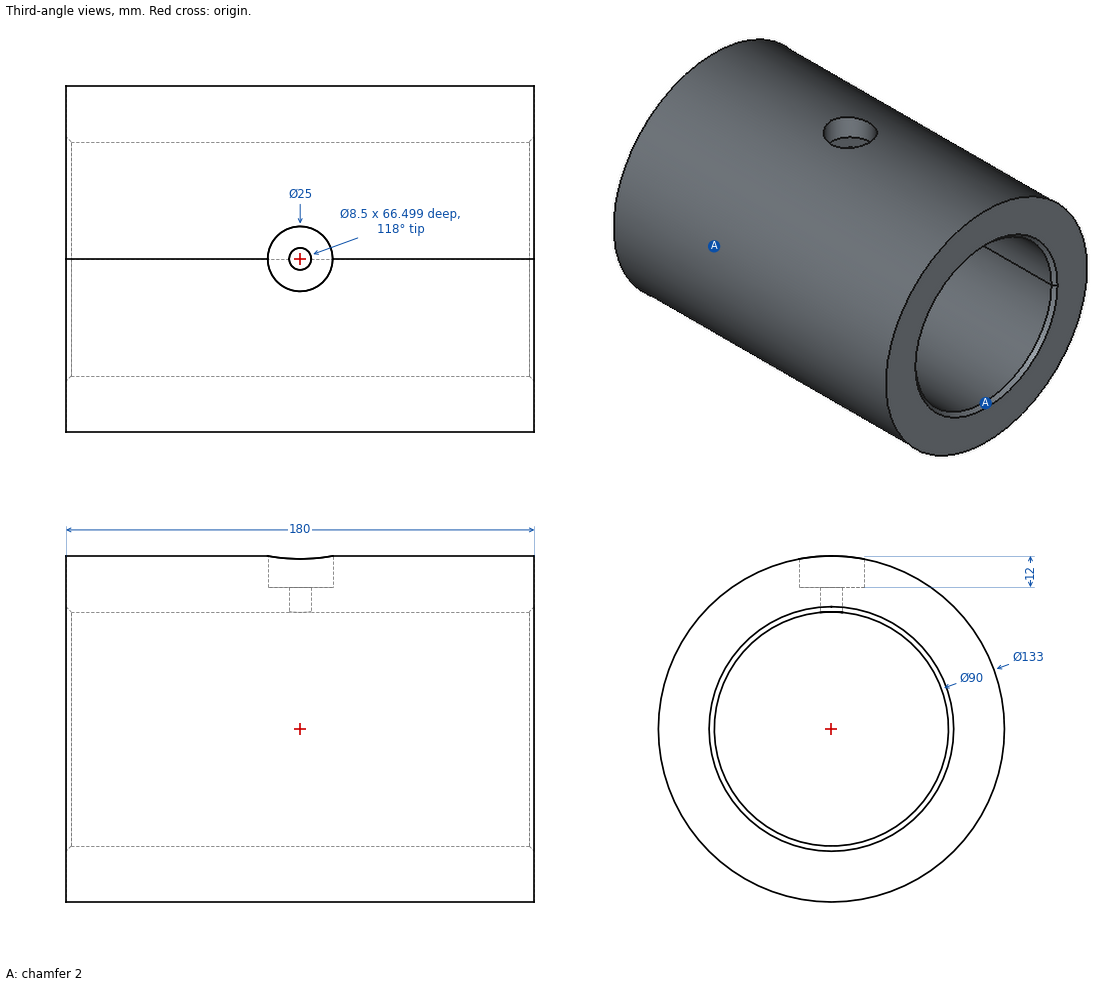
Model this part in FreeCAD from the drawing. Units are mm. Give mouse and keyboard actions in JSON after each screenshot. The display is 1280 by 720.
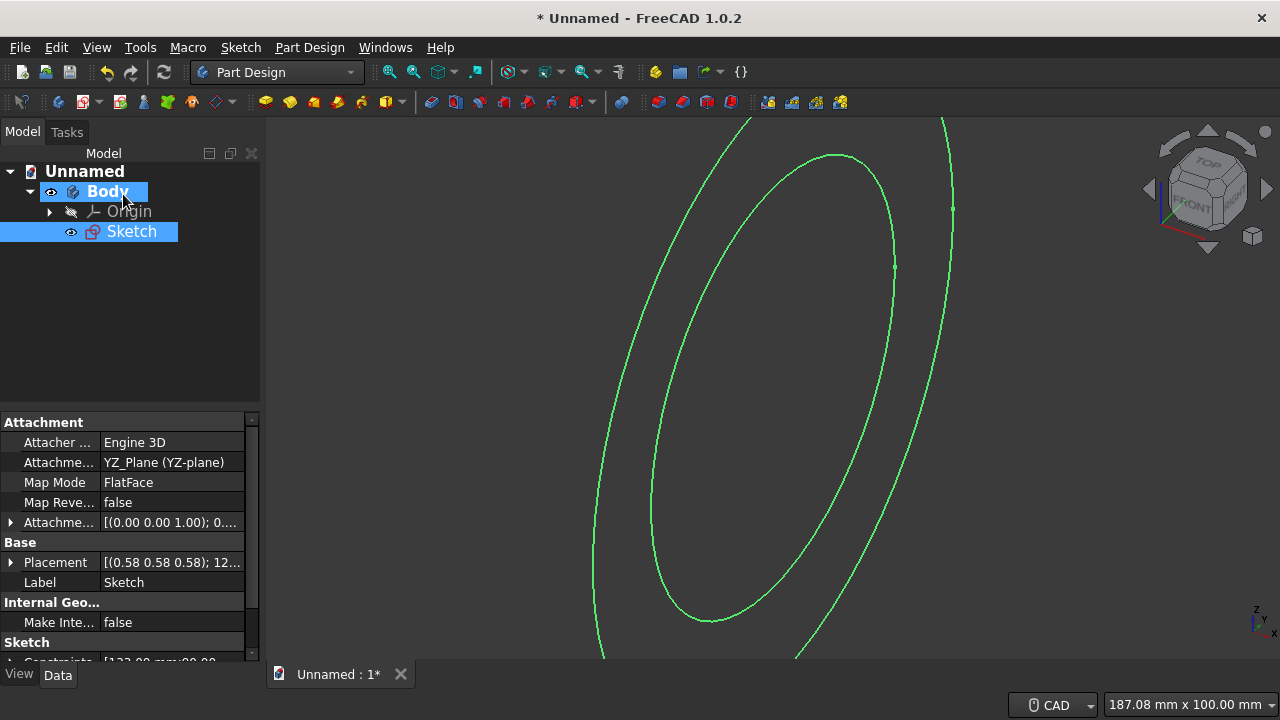
{"action": "left_click", "coordinate": [266, 102]}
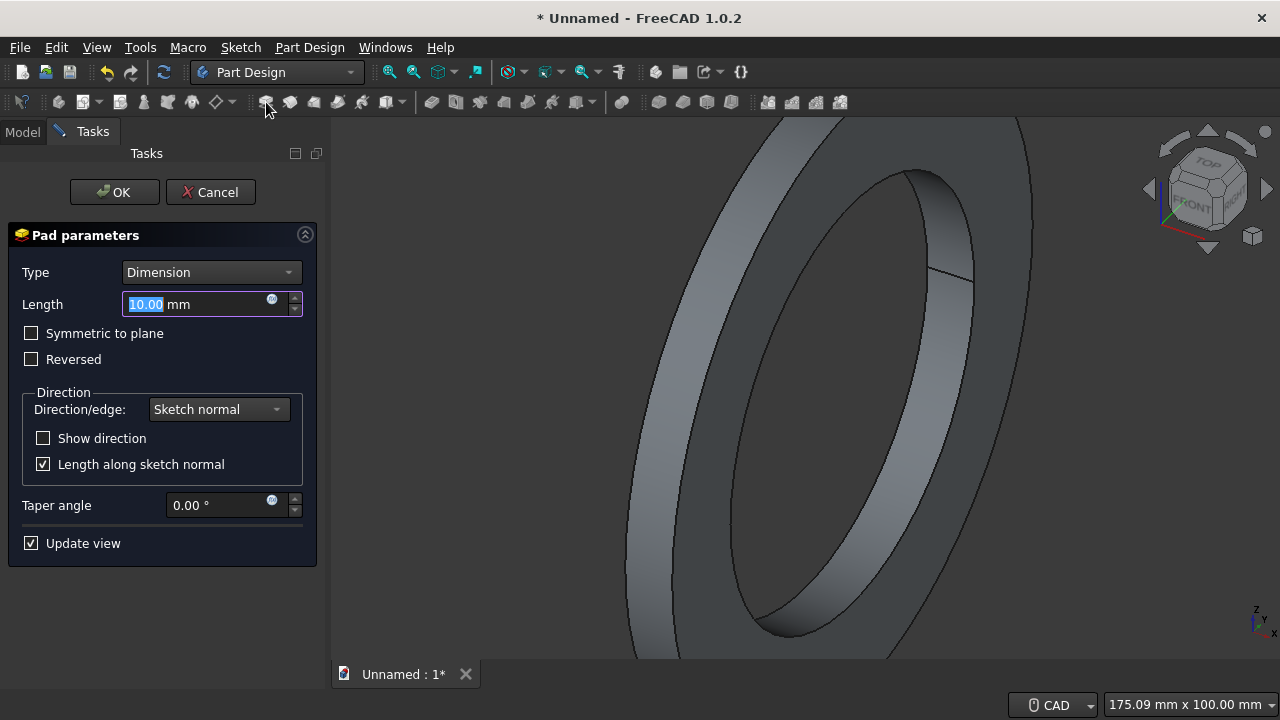
{"action": "type", "text": "180"}
{"action": "key", "text": "Tab"}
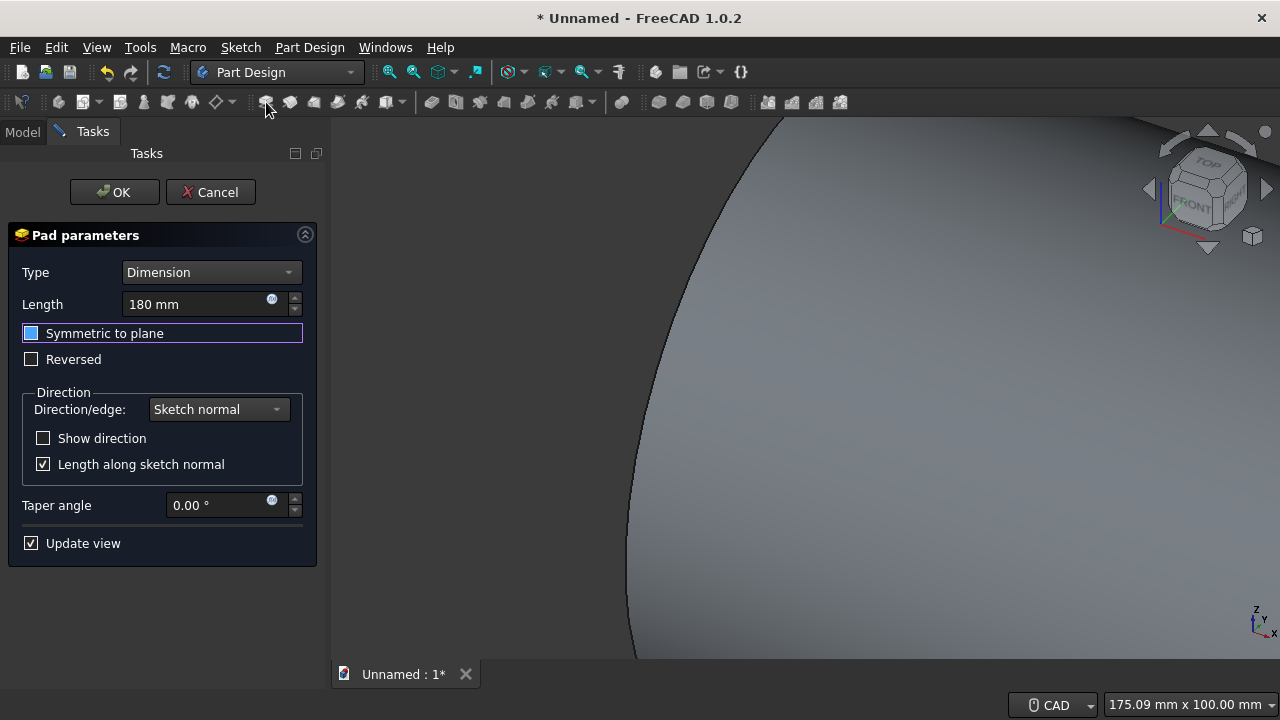
{"action": "left_click", "coordinate": [30, 333]}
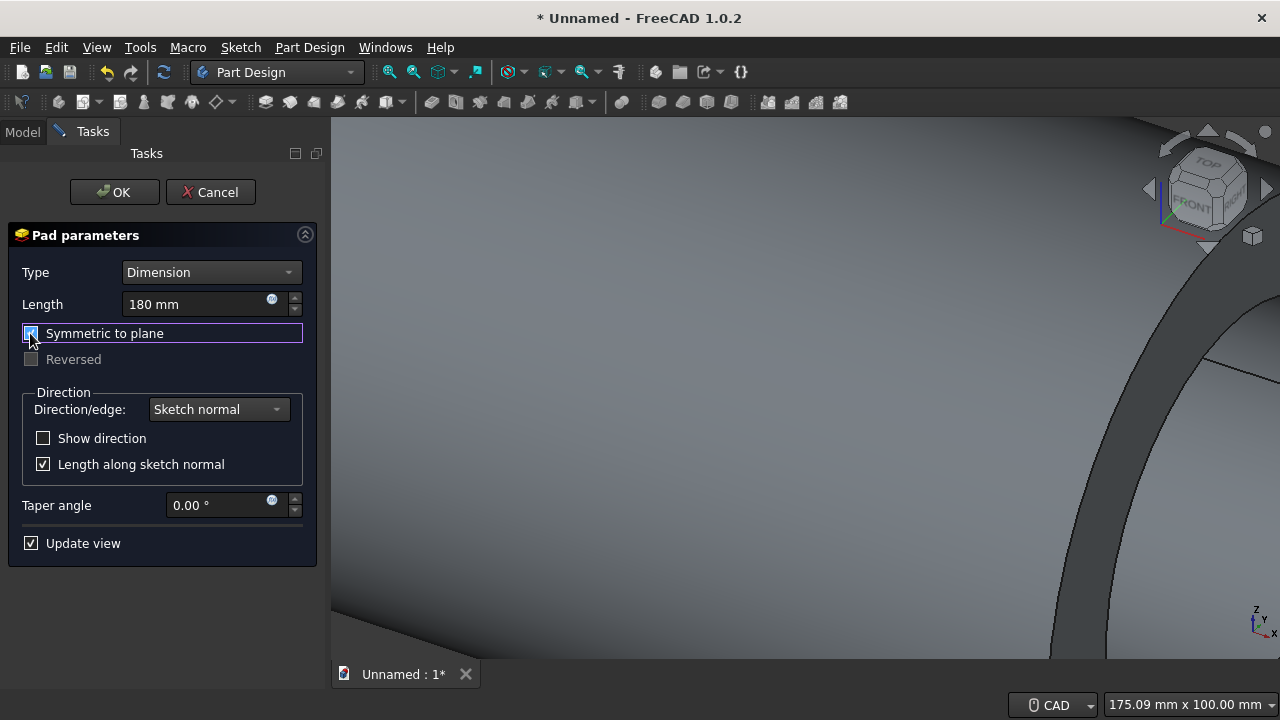
{"action": "left_click", "coordinate": [115, 192]}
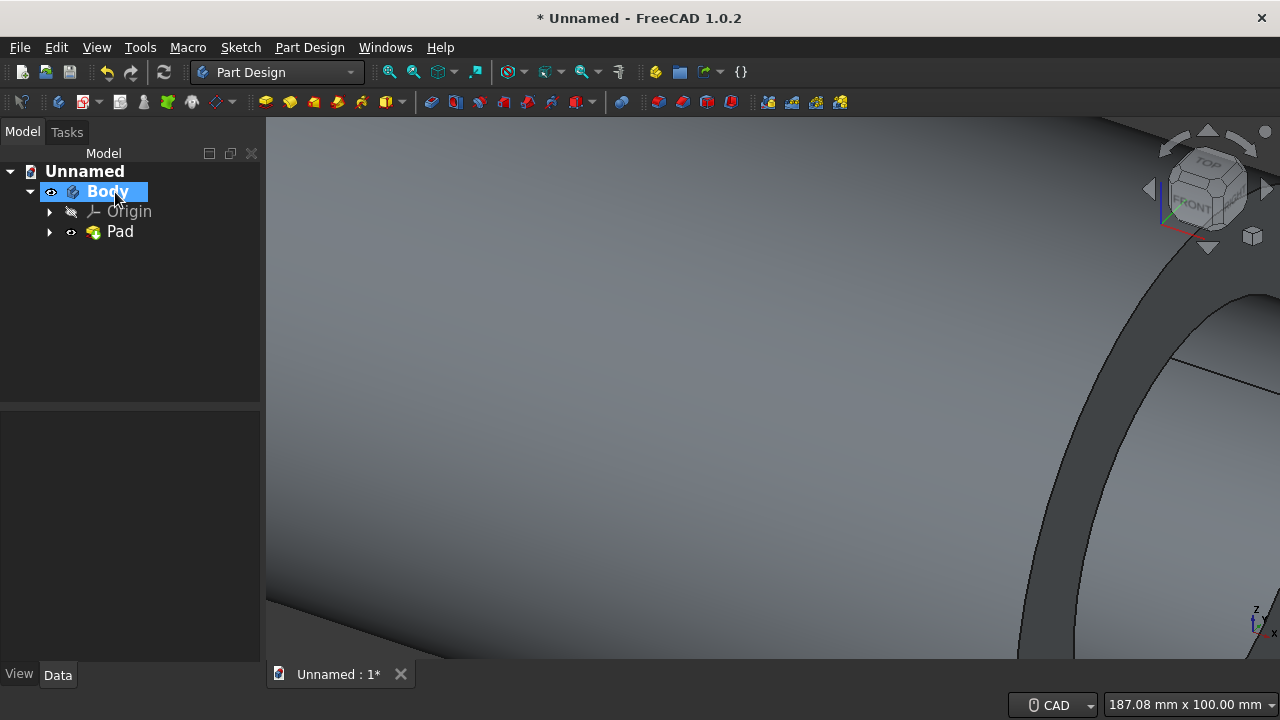
{"action": "left_click", "coordinate": [390, 72]}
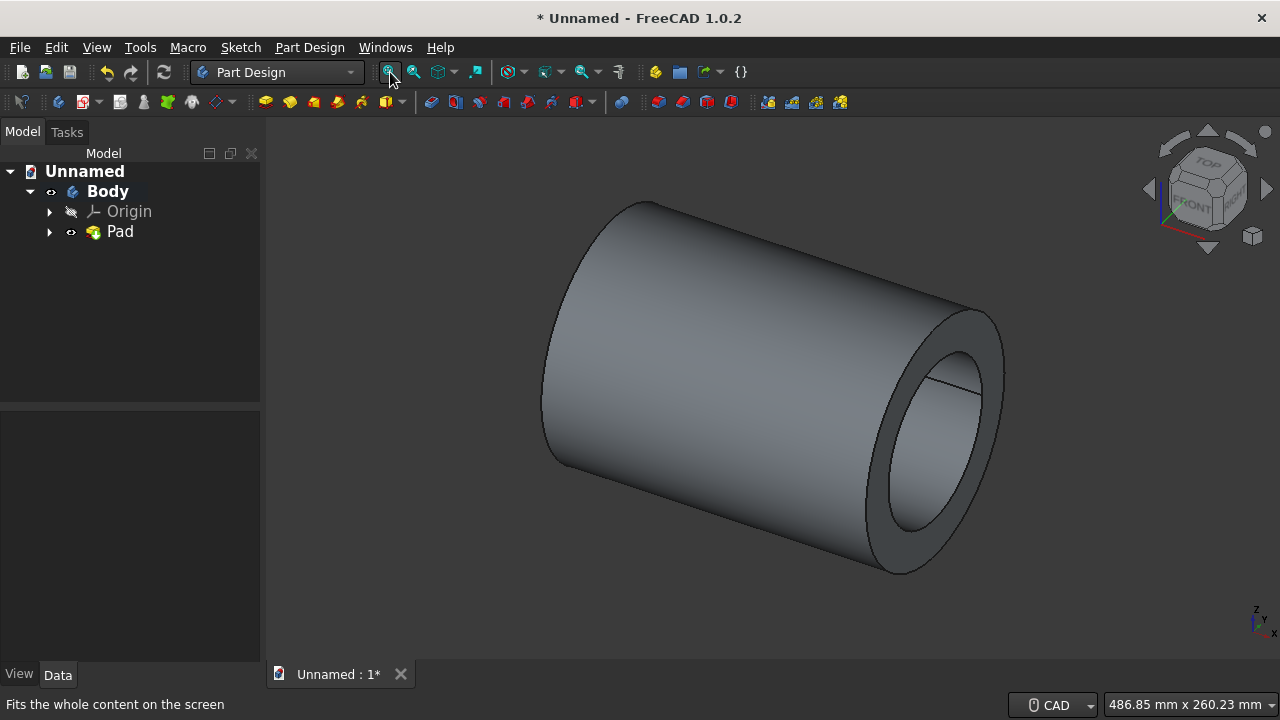
{"action": "left_click", "coordinate": [50, 212]}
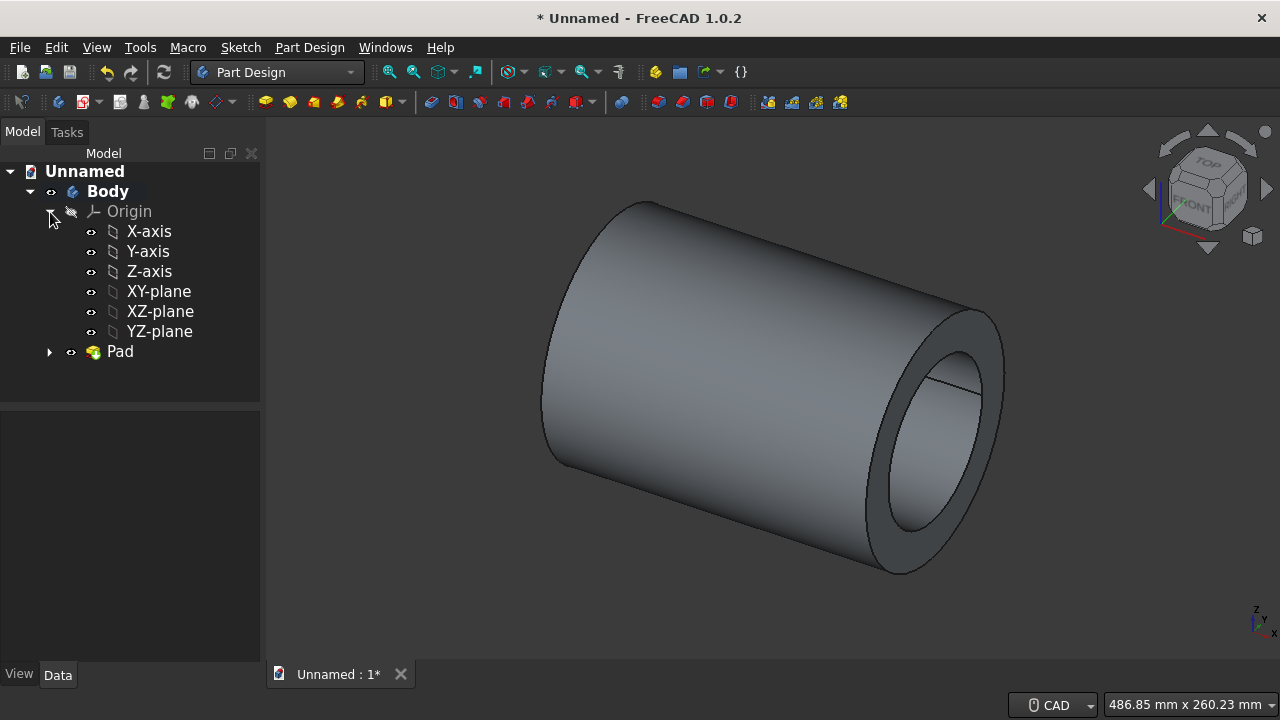
{"action": "left_click", "coordinate": [136, 292]}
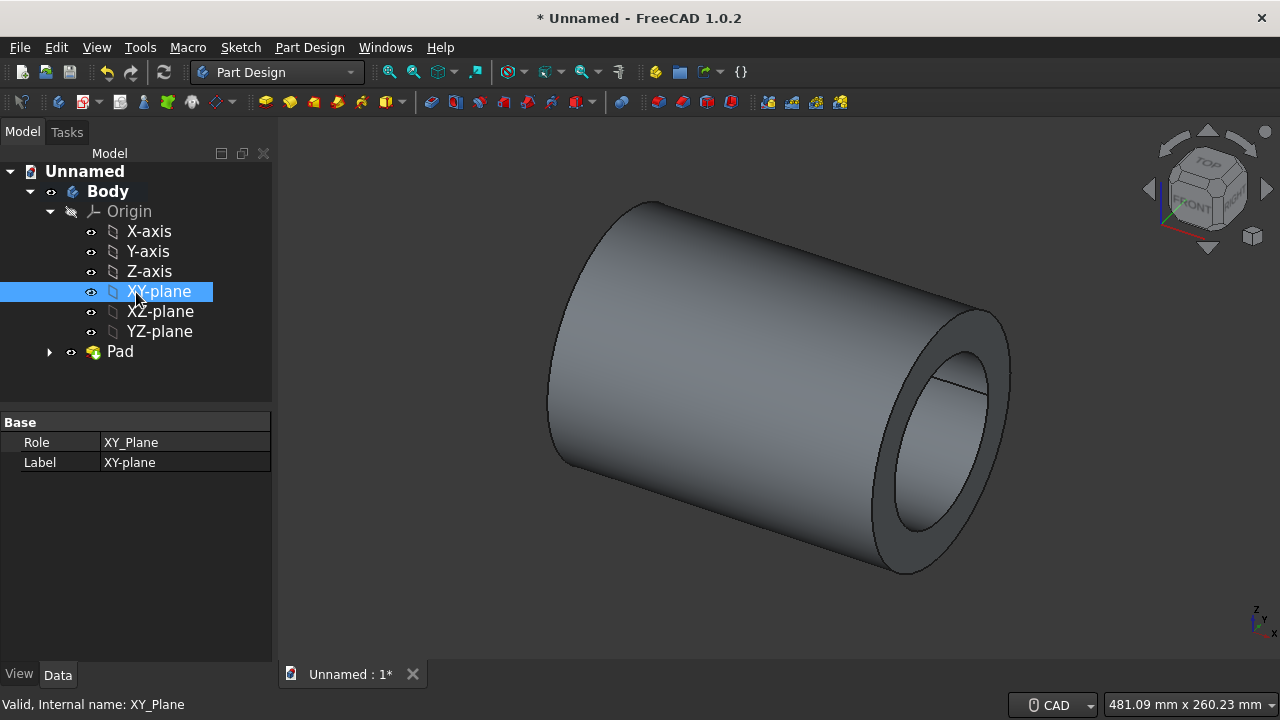
{"action": "left_click", "coordinate": [216, 102]}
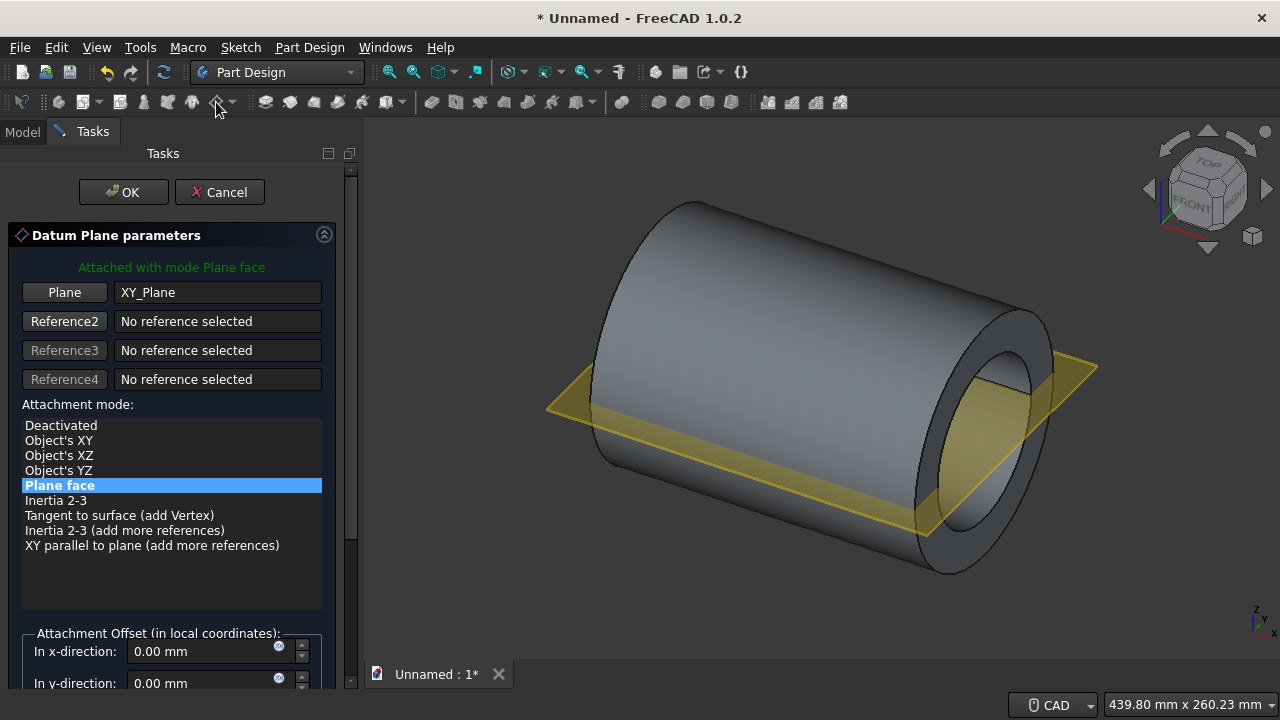
{"action": "scroll", "coordinate": [351, 426], "scroll_direction": "down", "scroll_amount": 2}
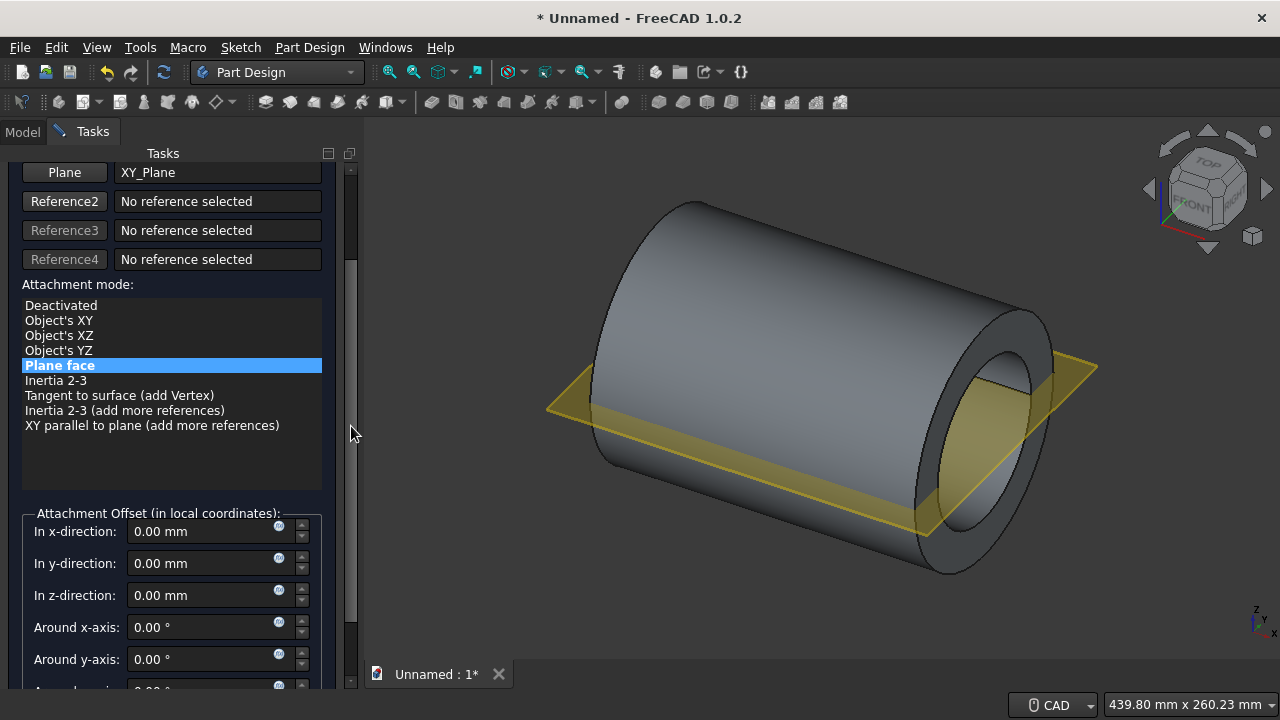
{"action": "triple_click", "coordinate": [210, 595]}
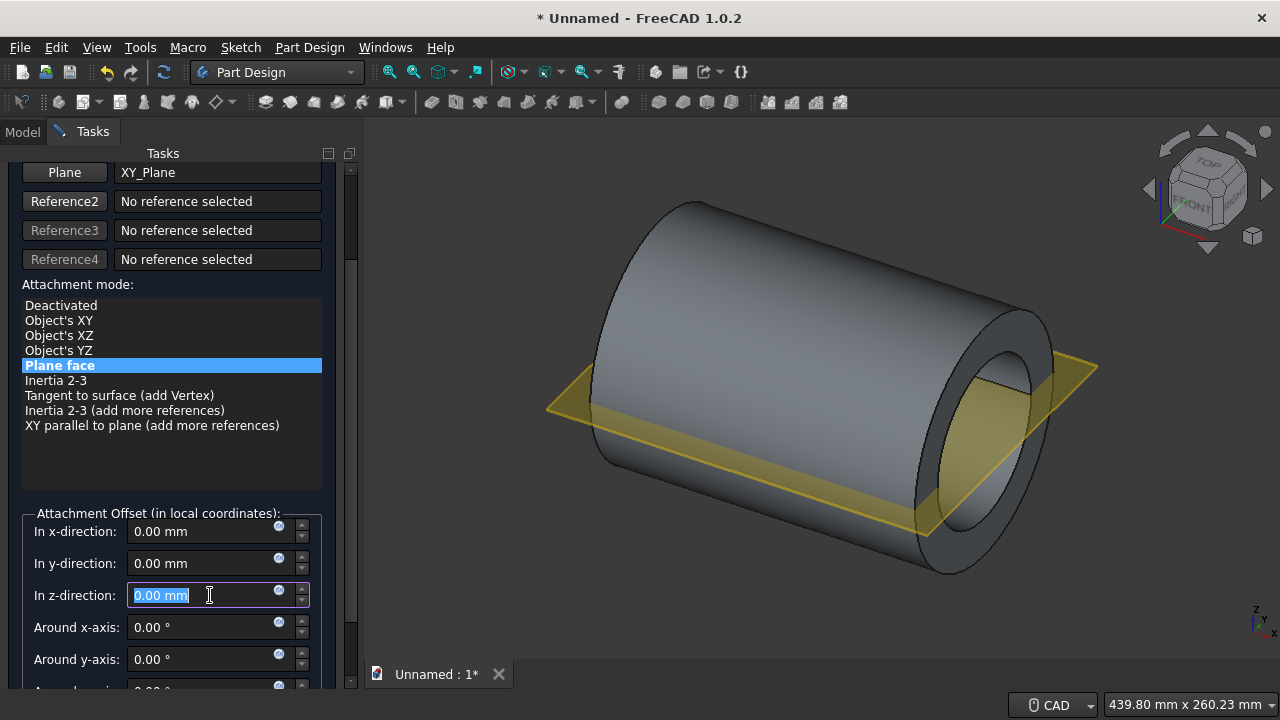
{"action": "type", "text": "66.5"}
{"action": "key", "text": "Tab"}